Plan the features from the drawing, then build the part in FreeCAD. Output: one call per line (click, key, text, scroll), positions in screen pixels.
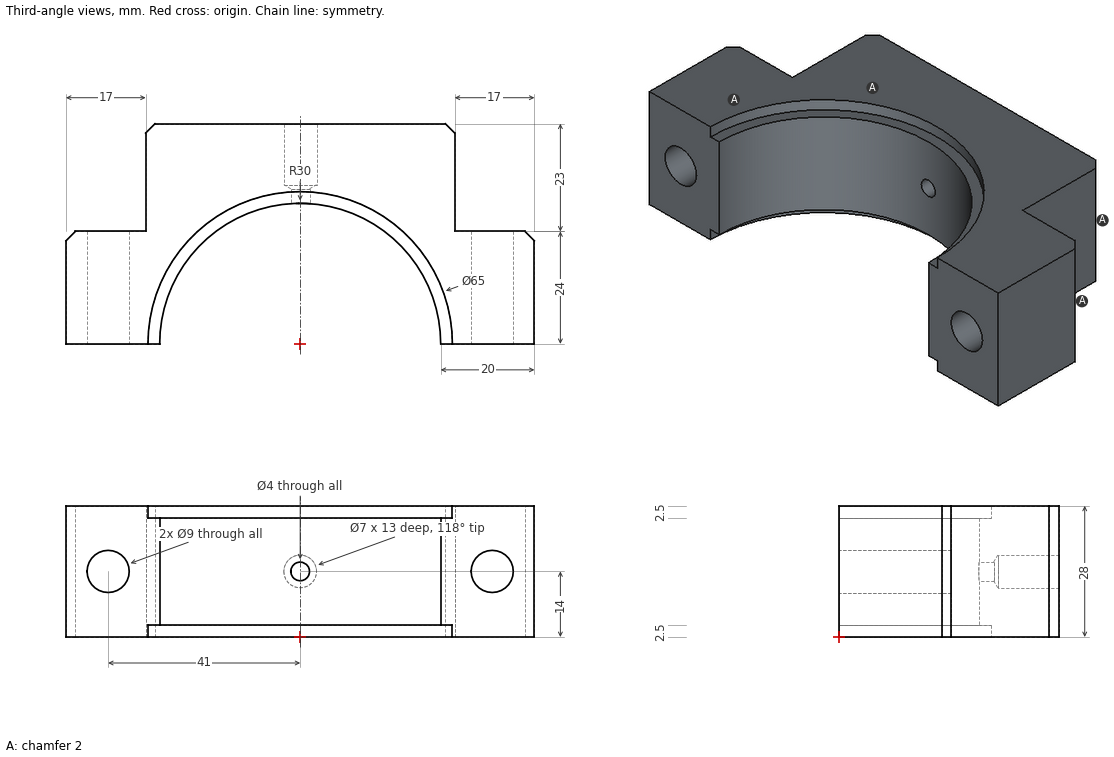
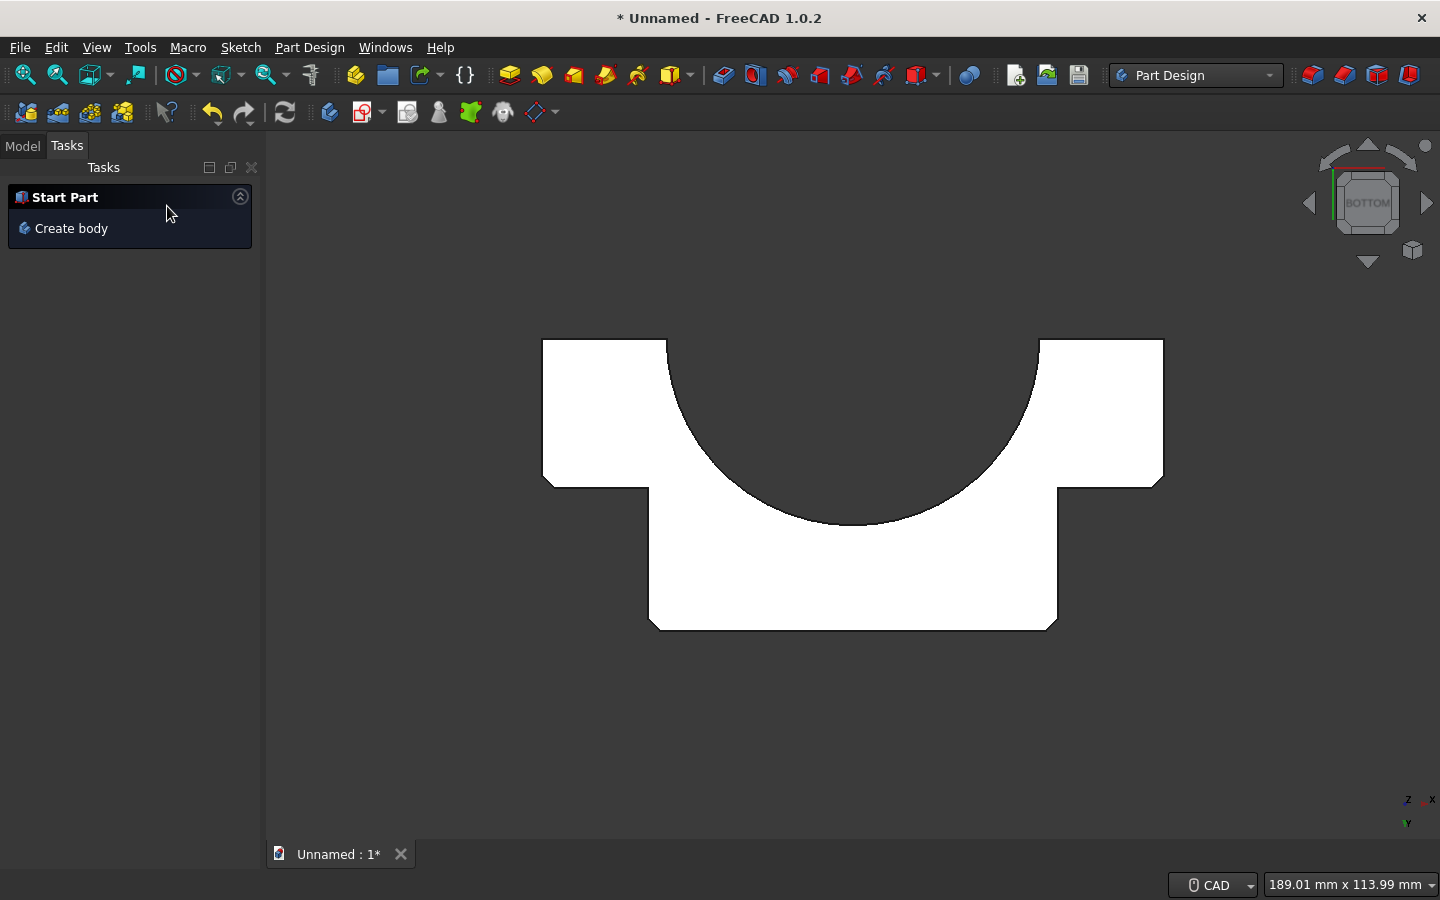
click(942, 567)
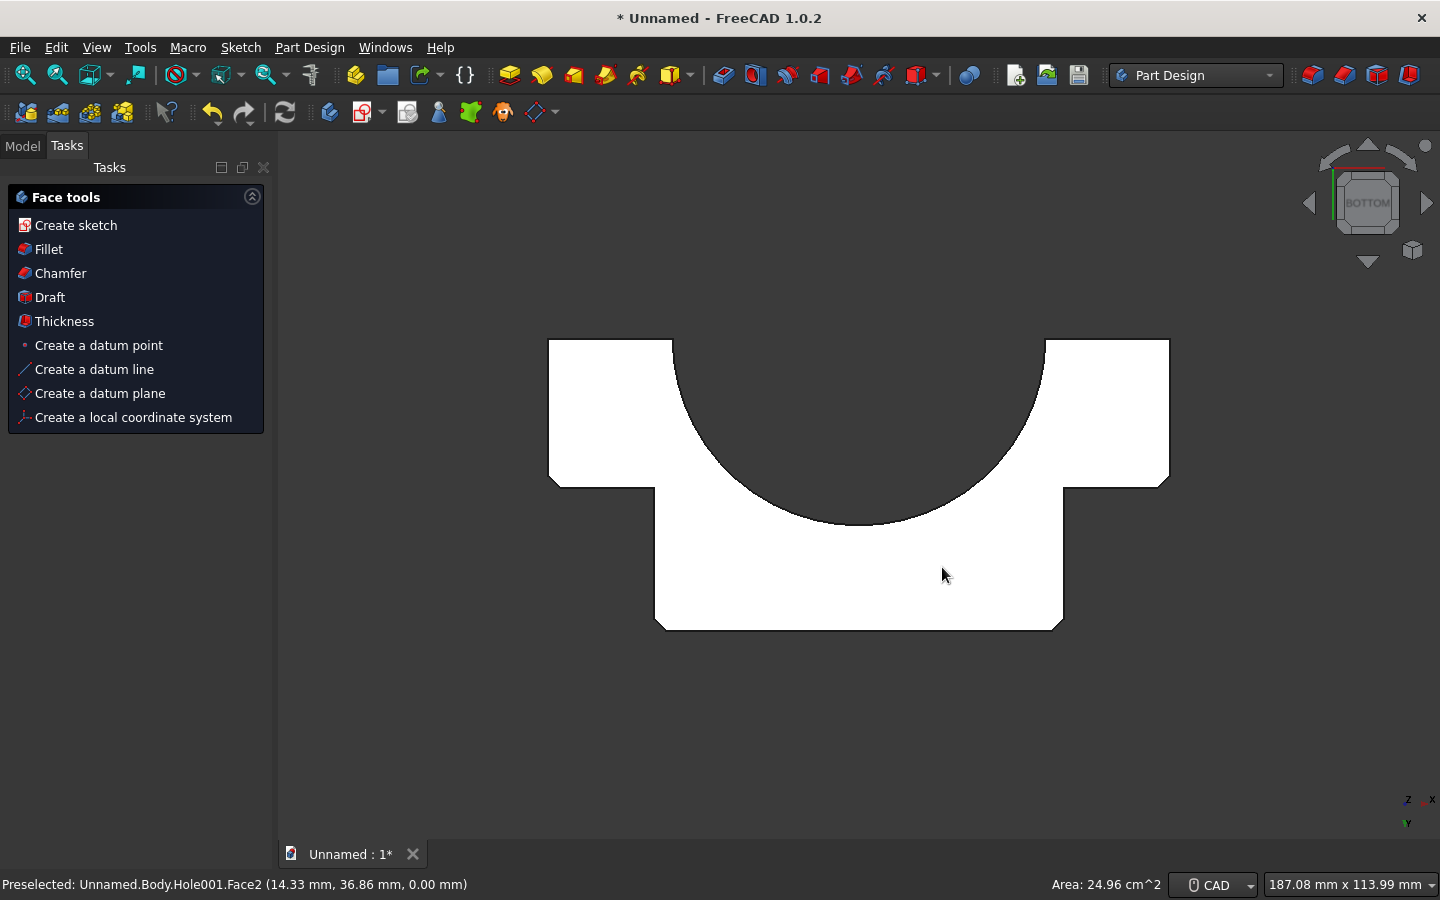
click(362, 112)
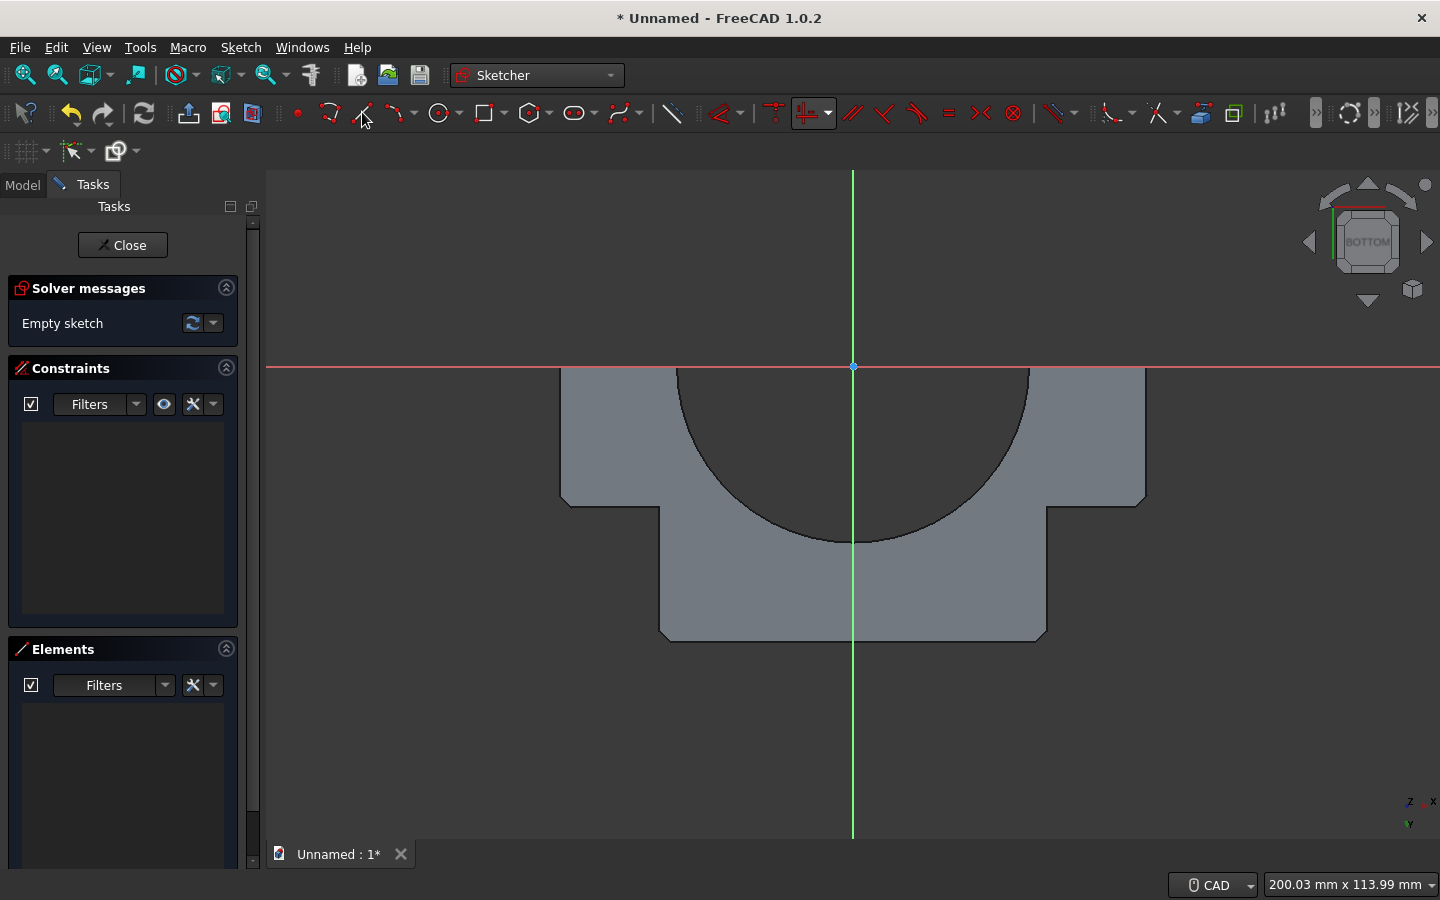
scroll(475, 811, down, 1)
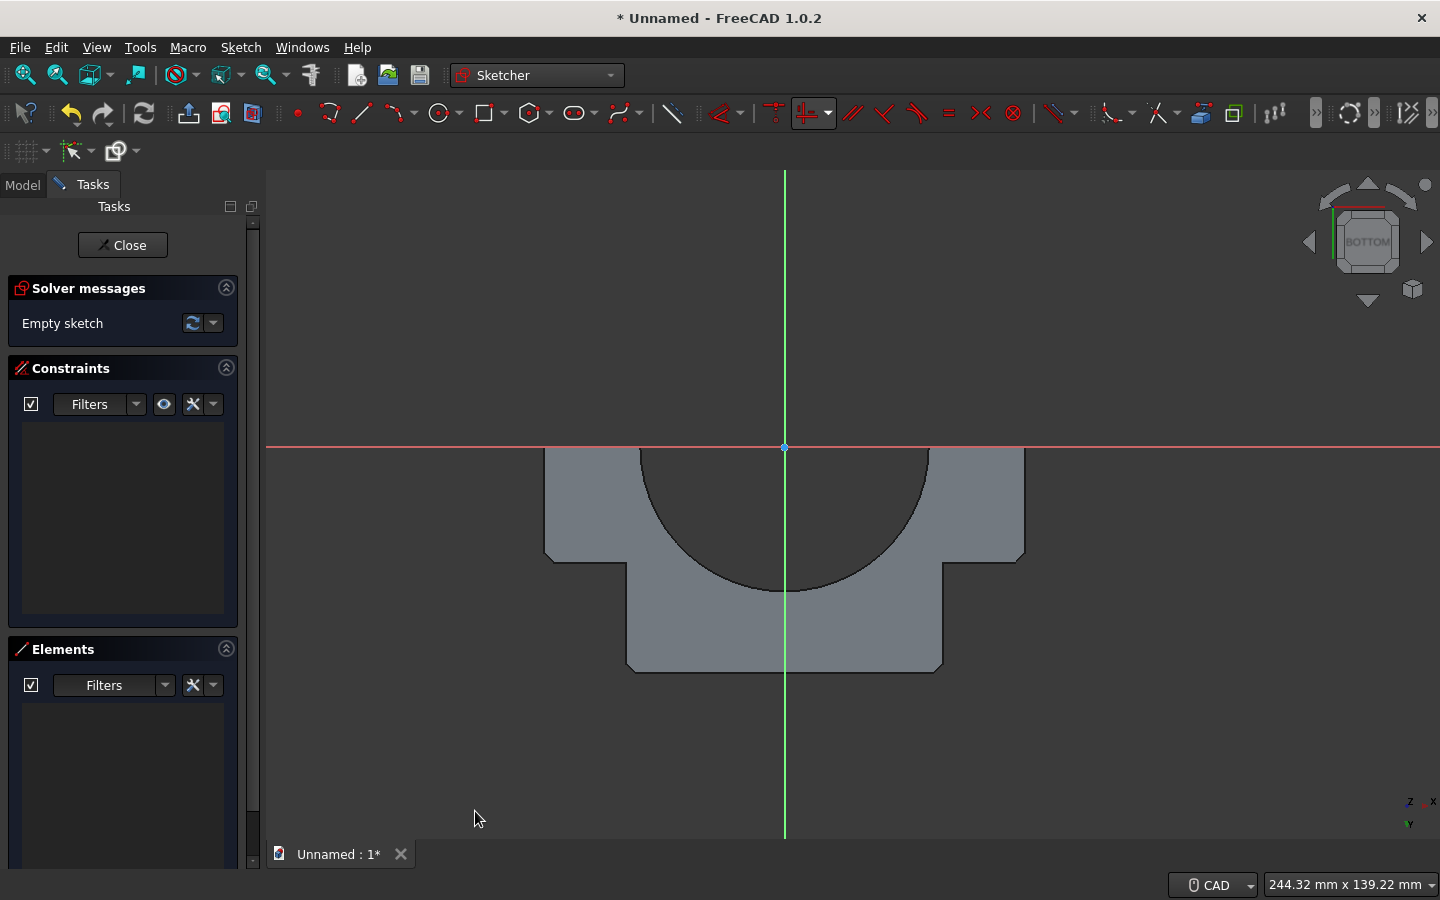
scroll(785, 331, up, 2)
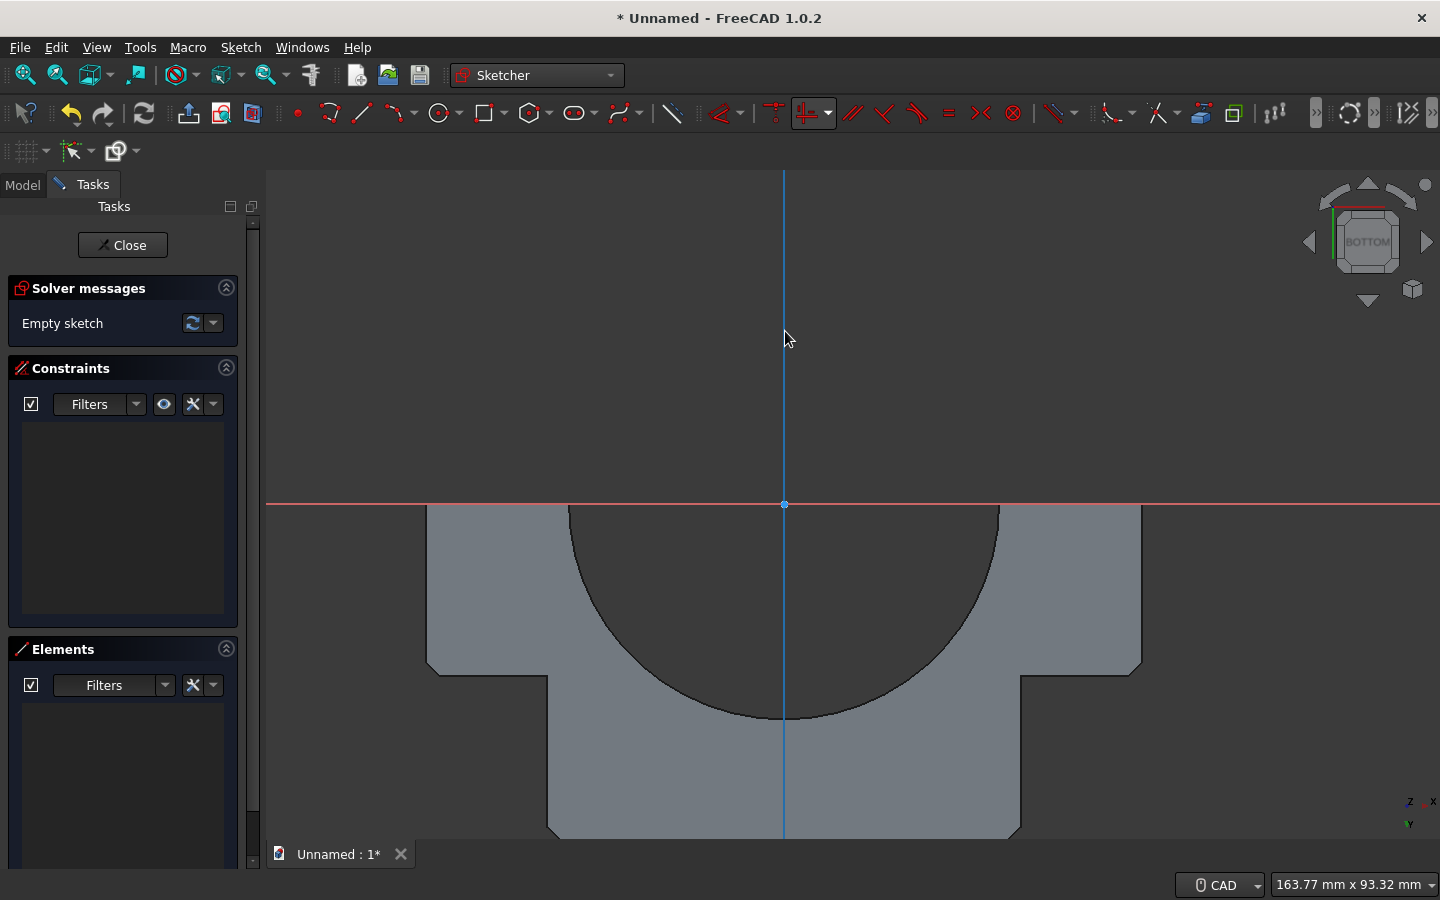
click(440, 114)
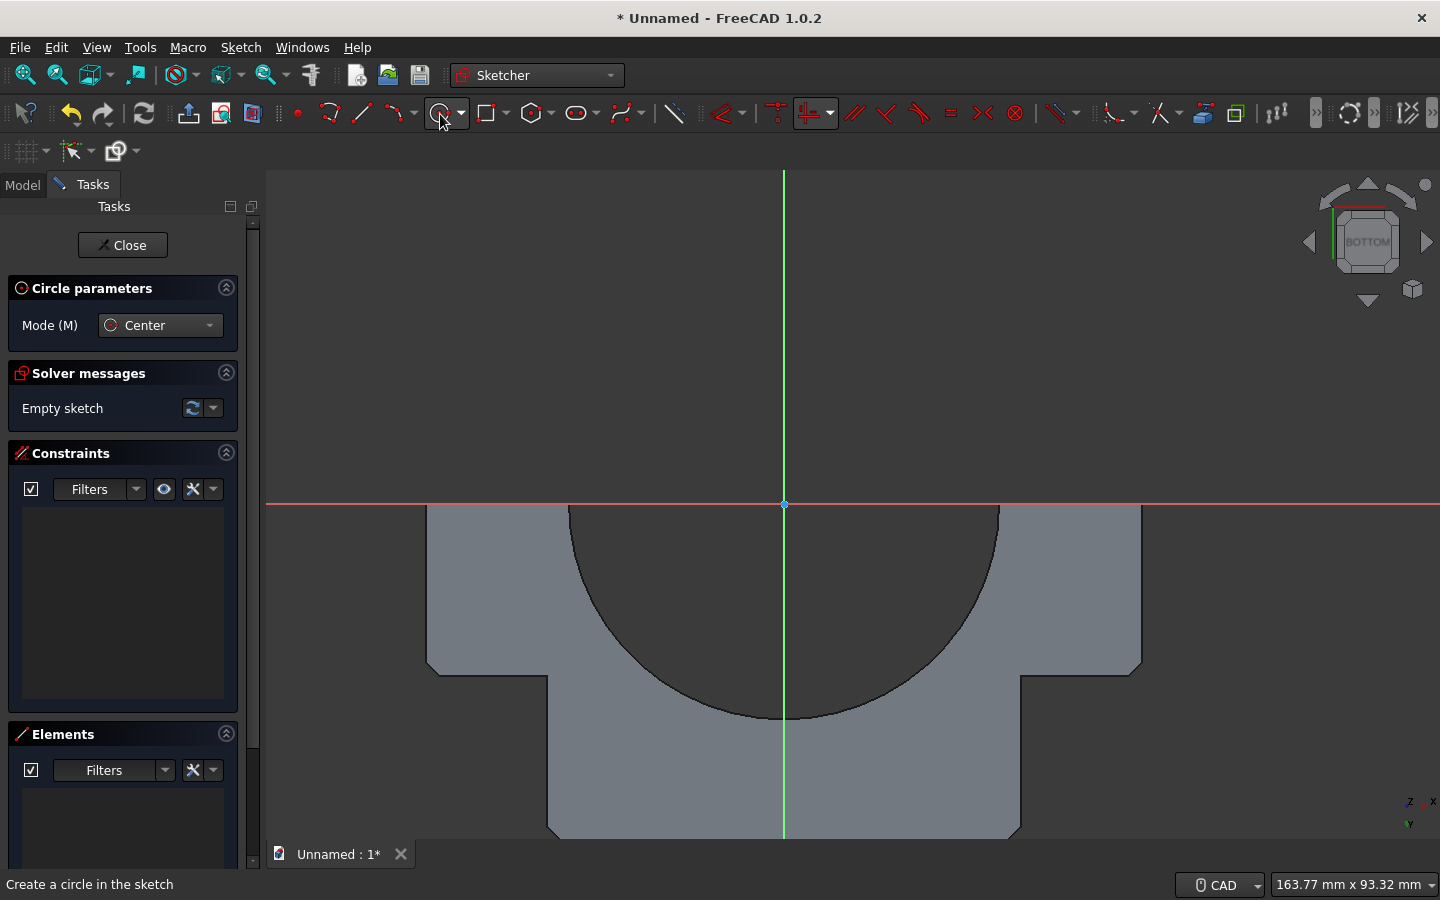
click(784, 504)
click(949, 340)
key(Escape)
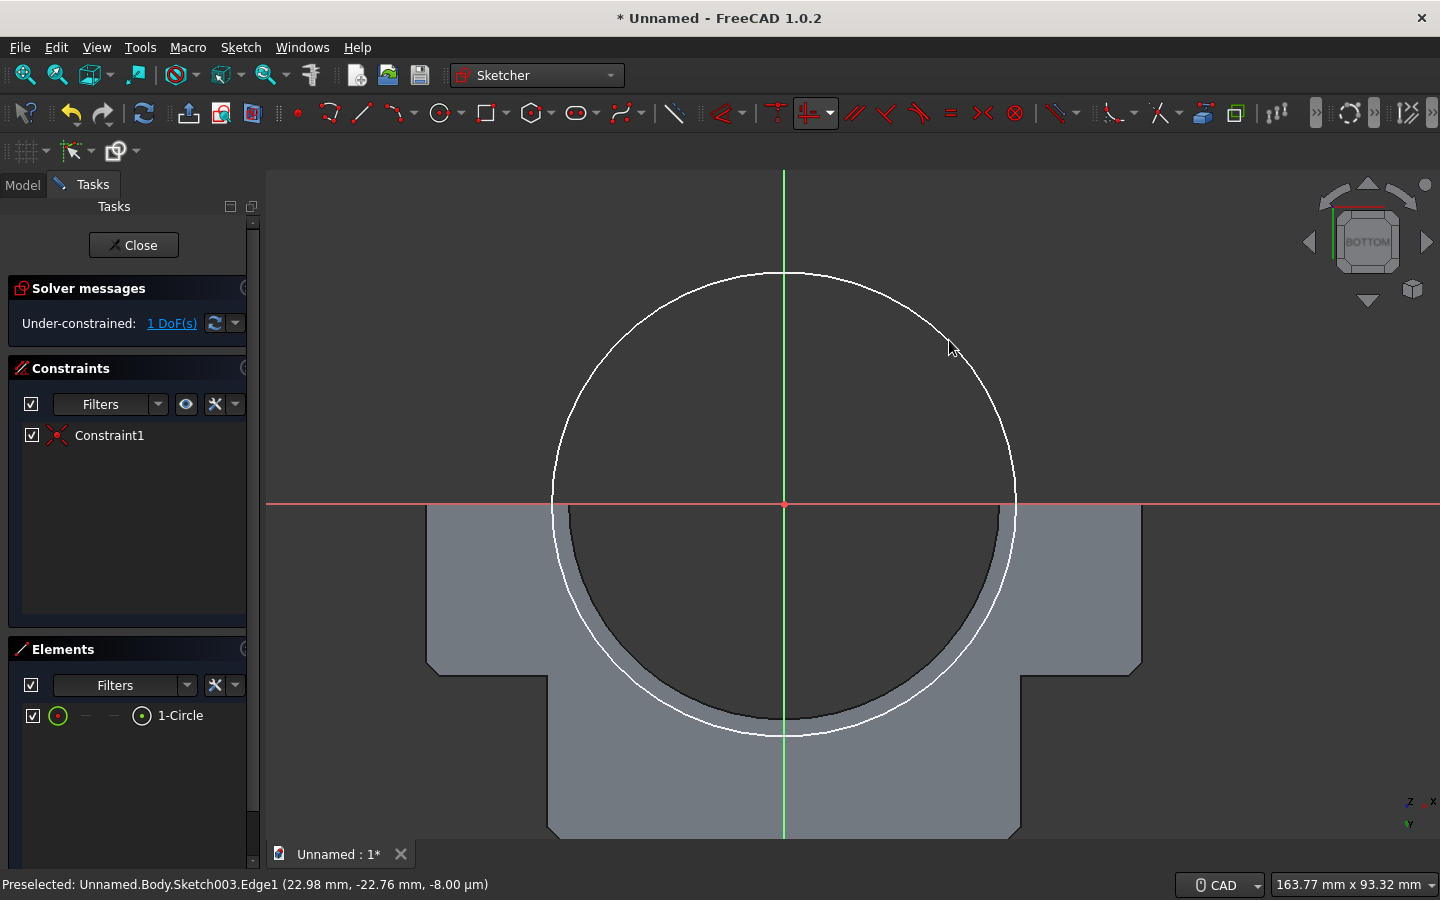
click(722, 114)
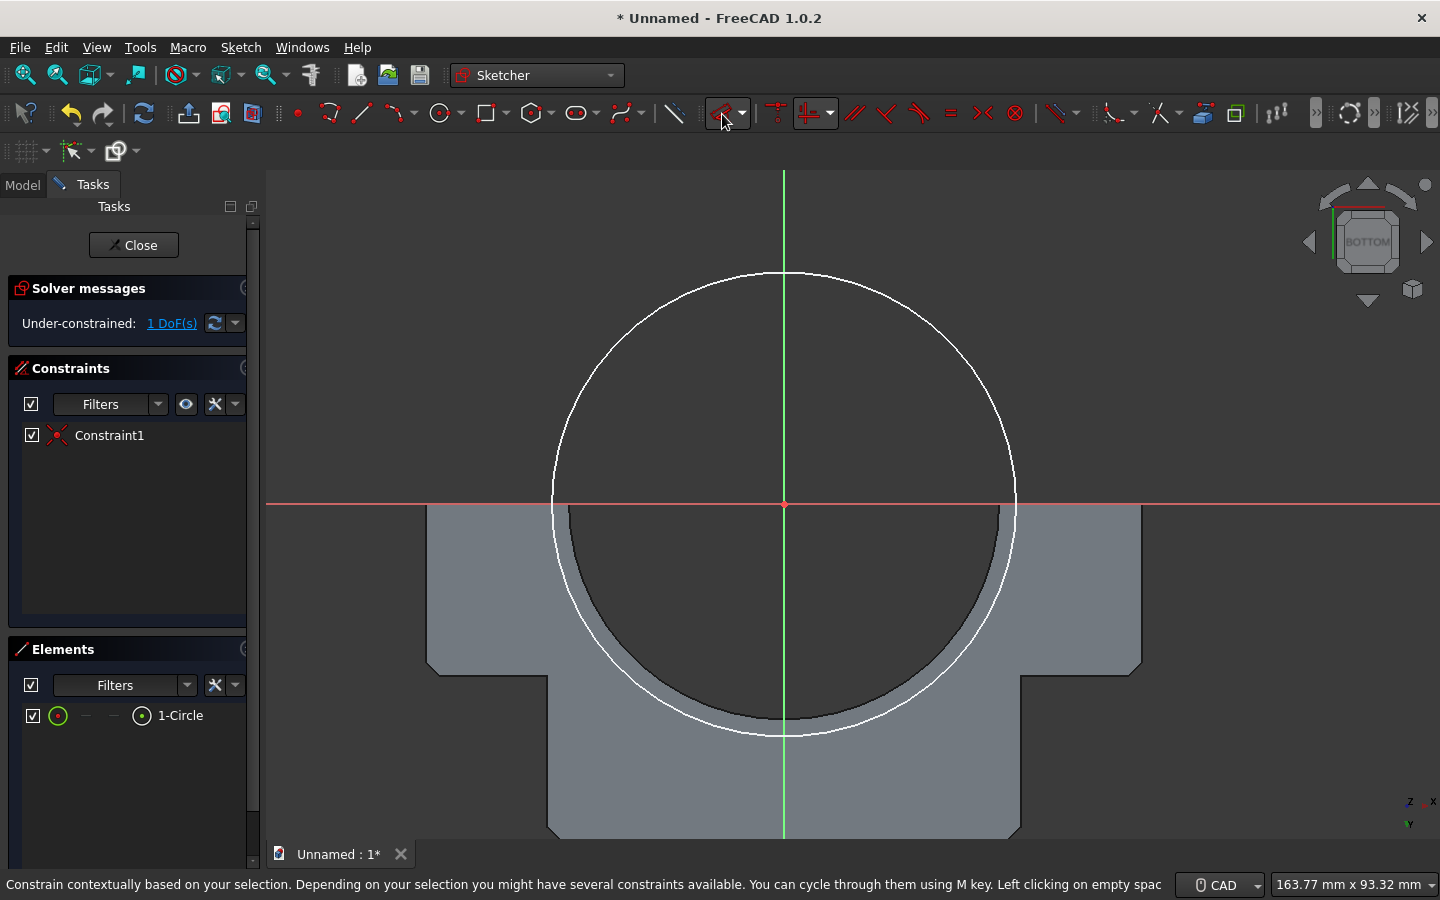
click(948, 340)
click(971, 317)